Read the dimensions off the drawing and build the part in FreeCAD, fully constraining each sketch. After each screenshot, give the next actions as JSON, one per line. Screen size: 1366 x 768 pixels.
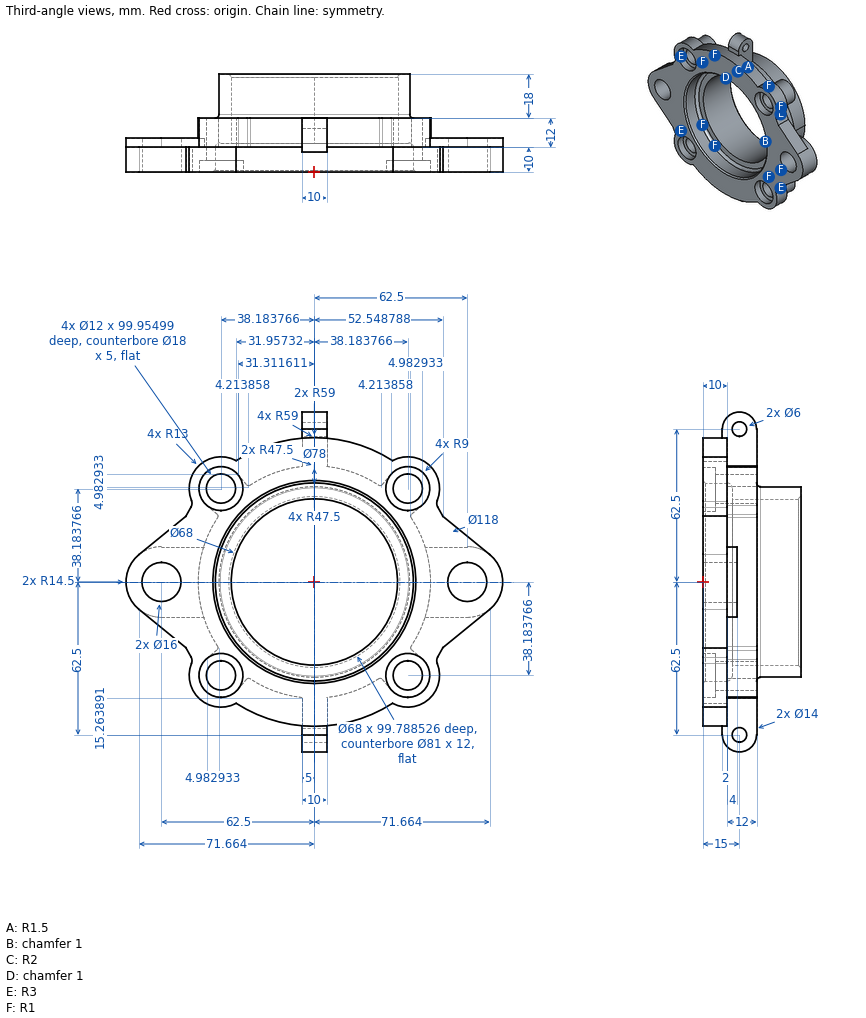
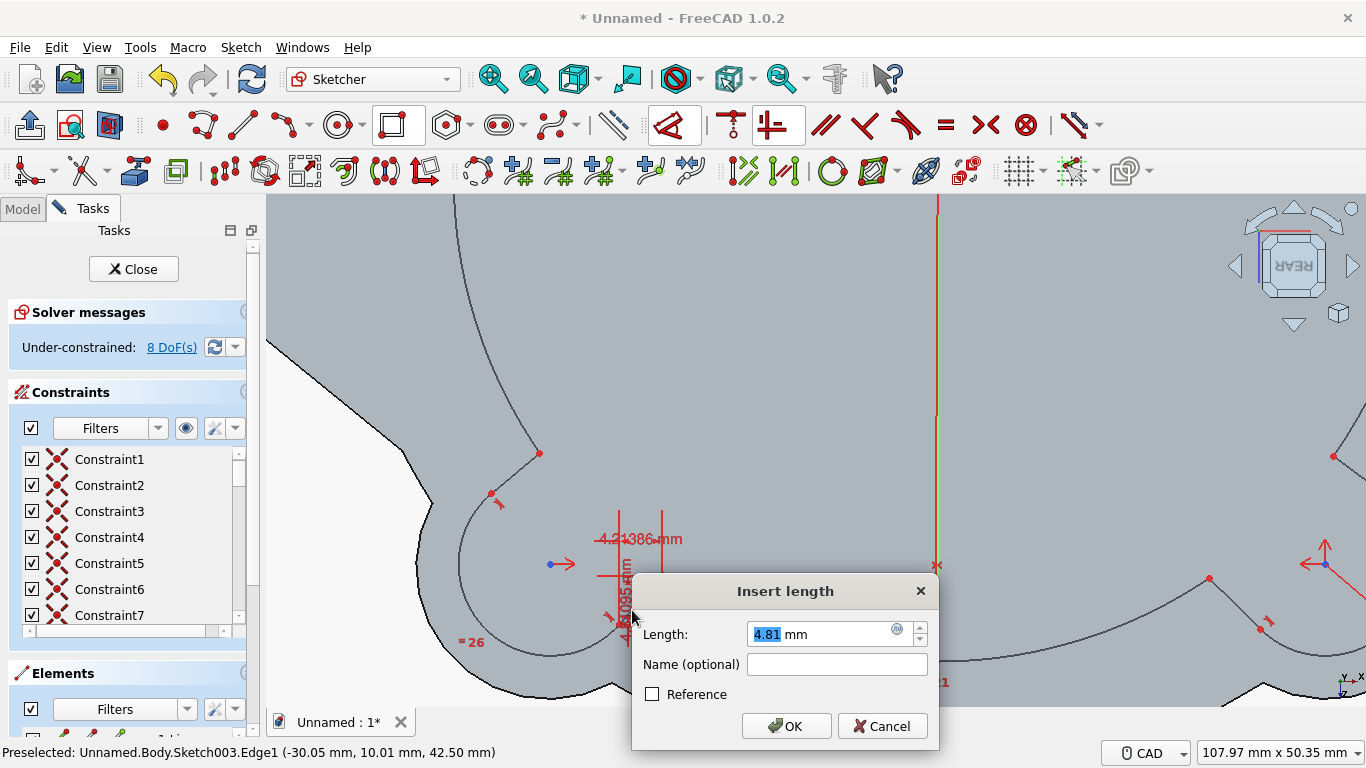
{"action": "type", "text": "4.982933"}
{"action": "key", "text": "Return"}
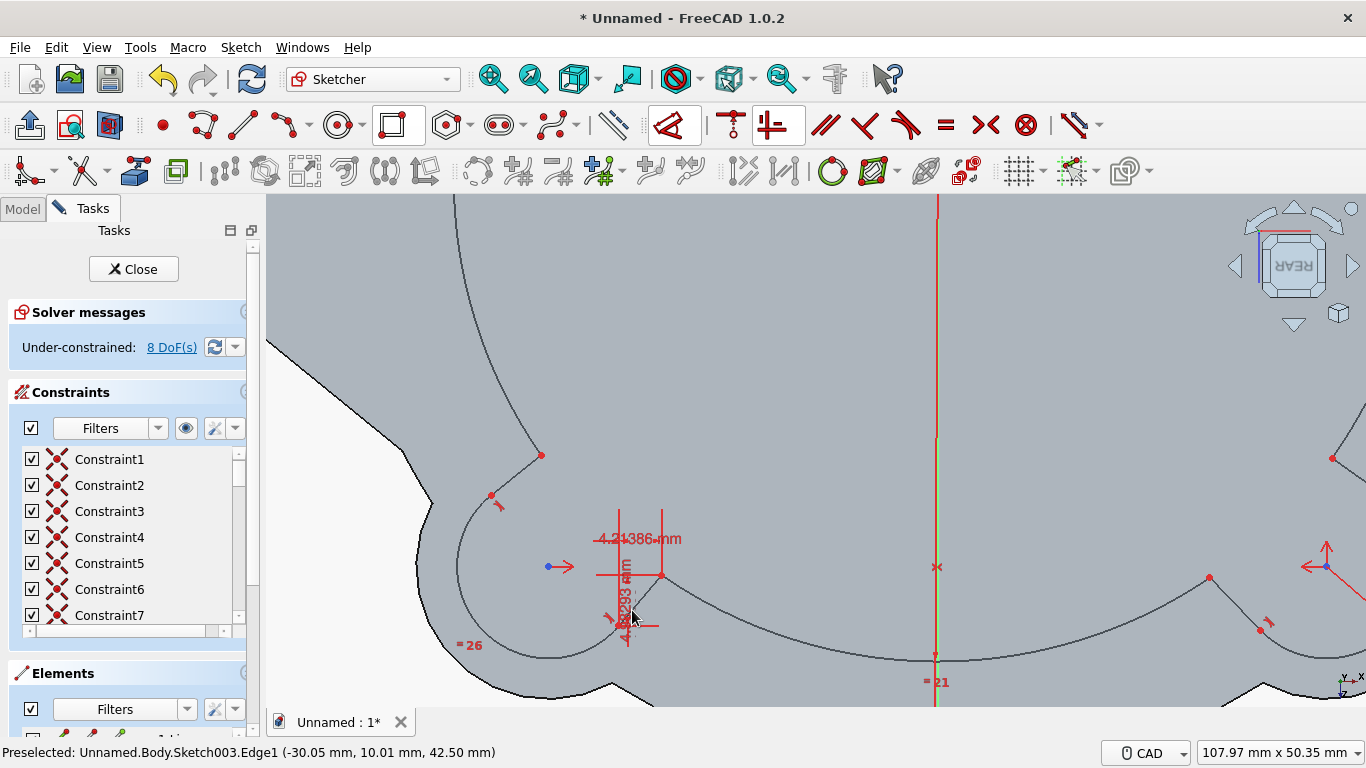
{"action": "scroll", "coordinate": [637, 609], "scroll_direction": "down", "scroll_amount": 5}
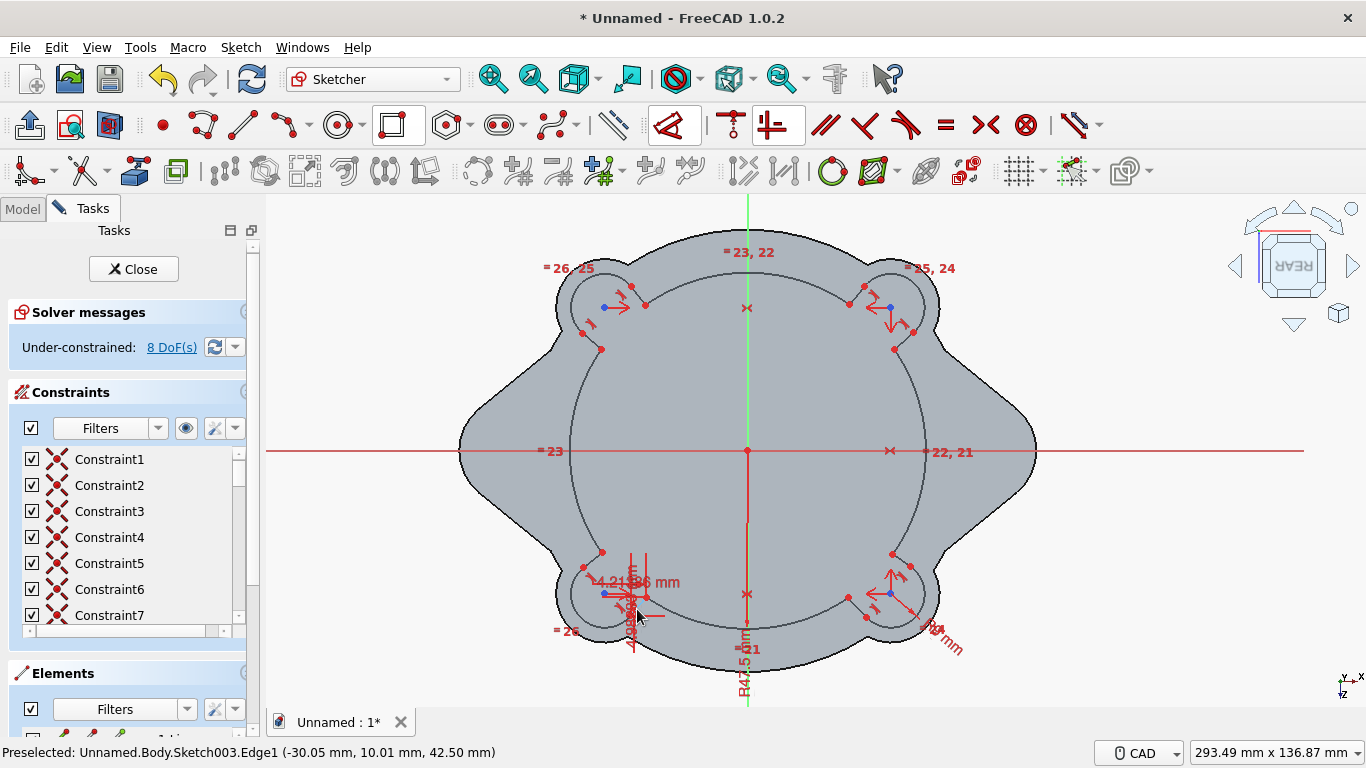
{"action": "scroll", "coordinate": [854, 604], "scroll_direction": "up", "scroll_amount": 5}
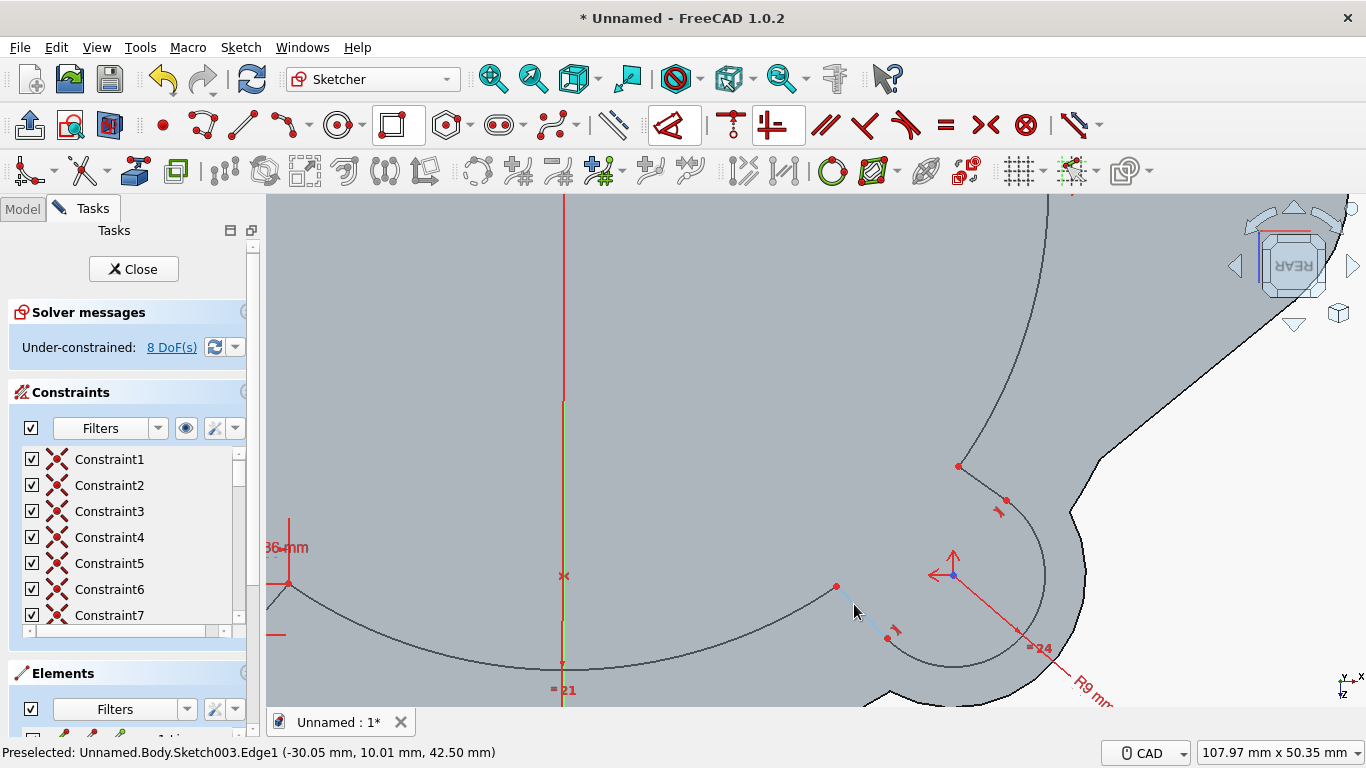
{"action": "left_click", "coordinate": [852, 602]}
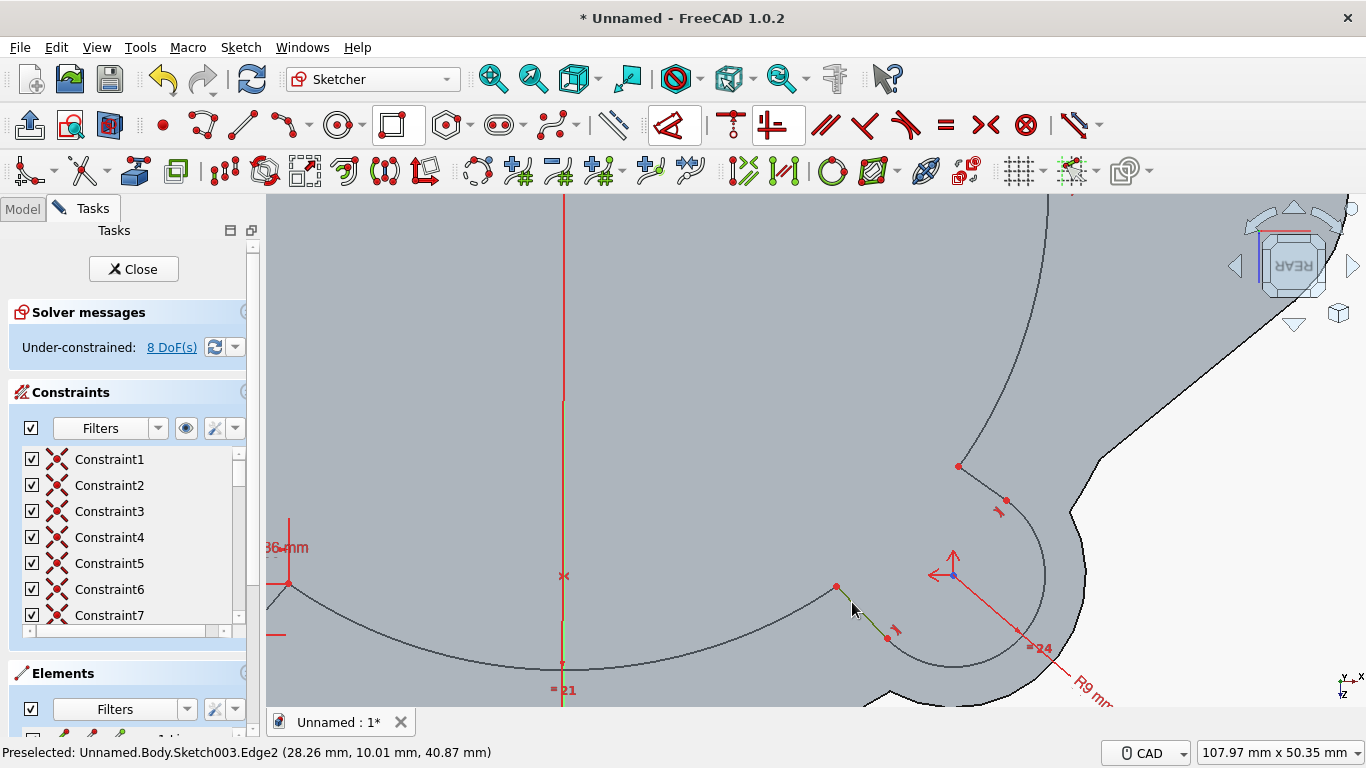
{"action": "left_click", "coordinate": [696, 126]}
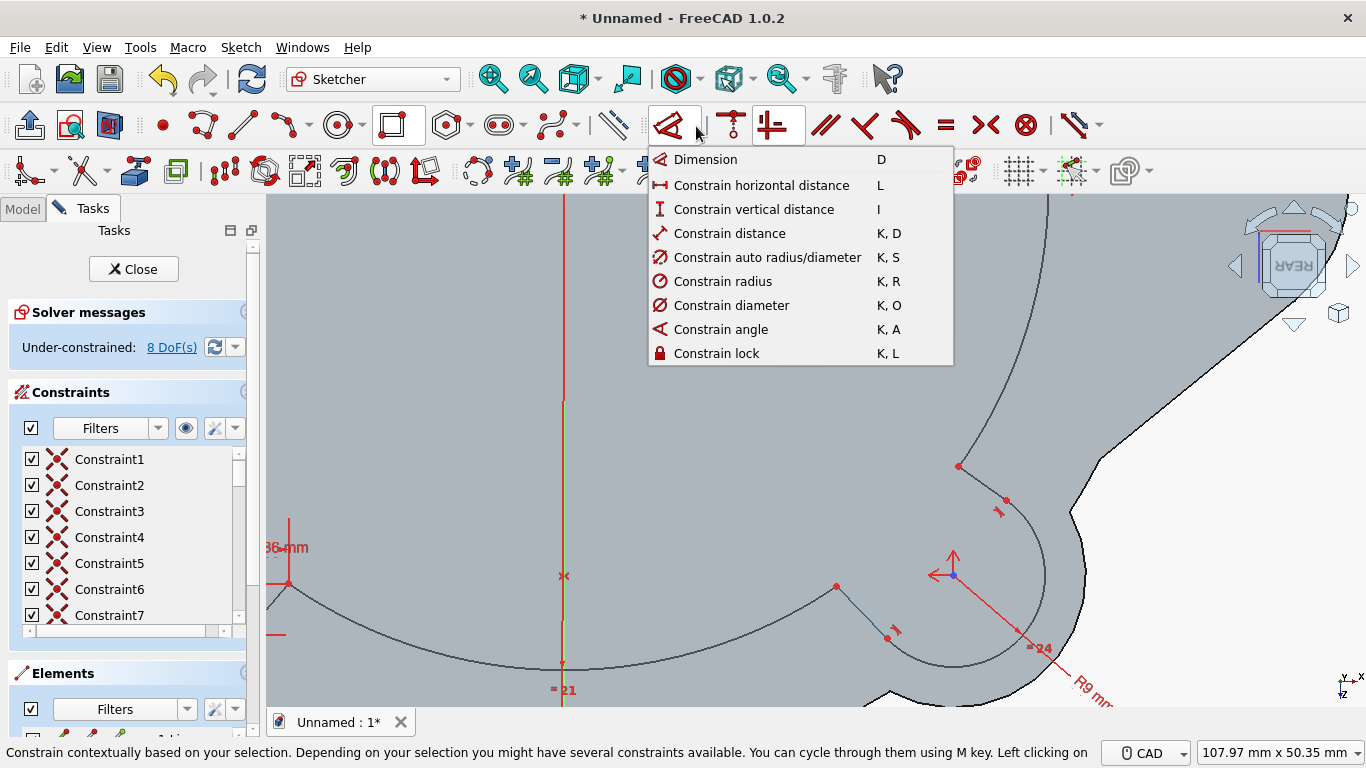
{"action": "left_click", "coordinate": [801, 185]}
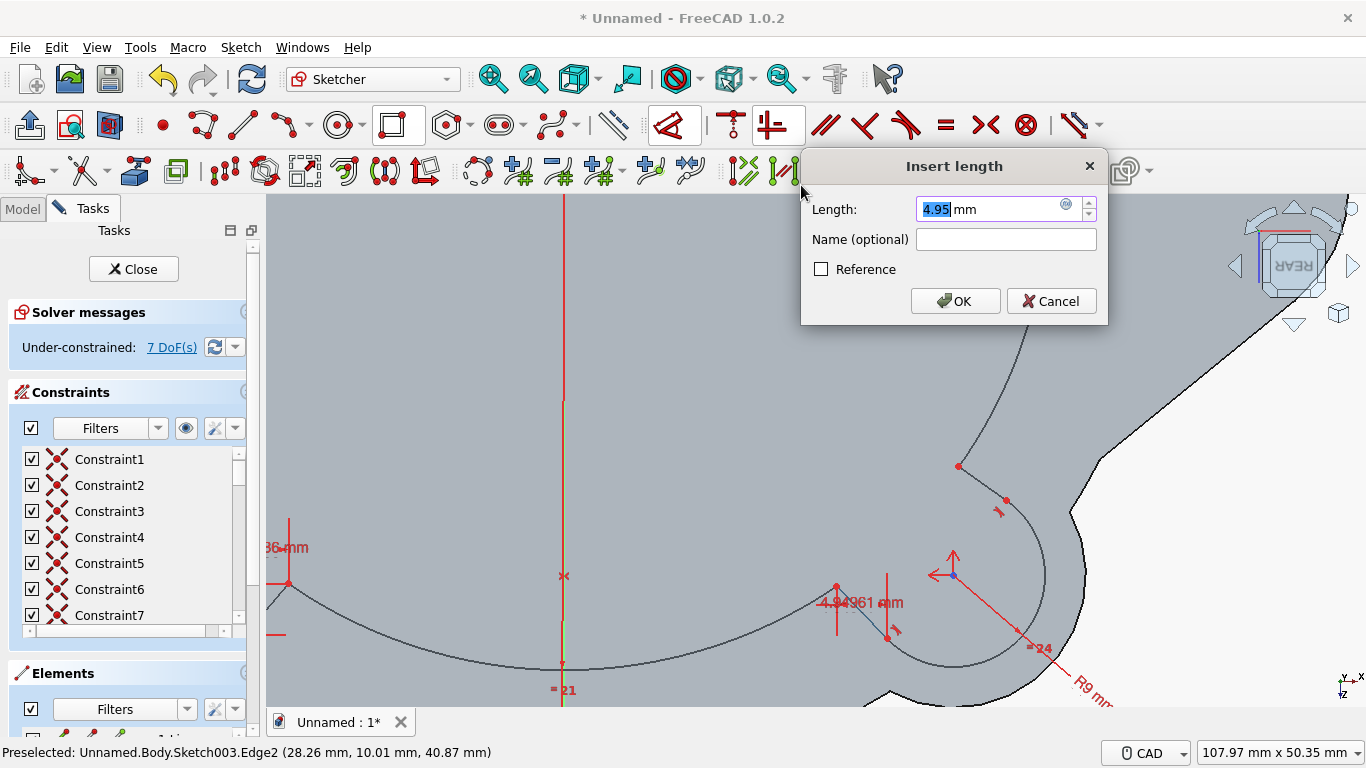
{"action": "type", "text": "4.213858"}
{"action": "key", "text": "Return"}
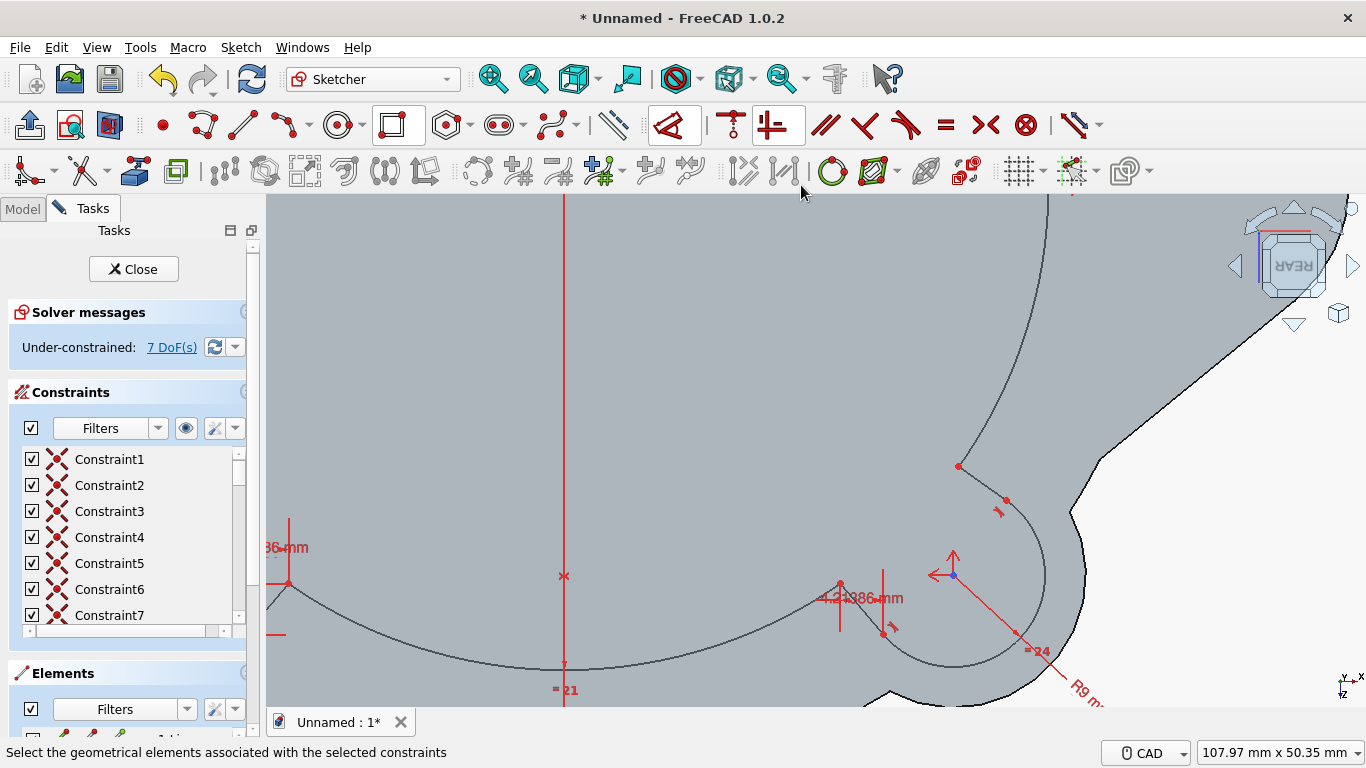
{"action": "left_click", "coordinate": [992, 490]}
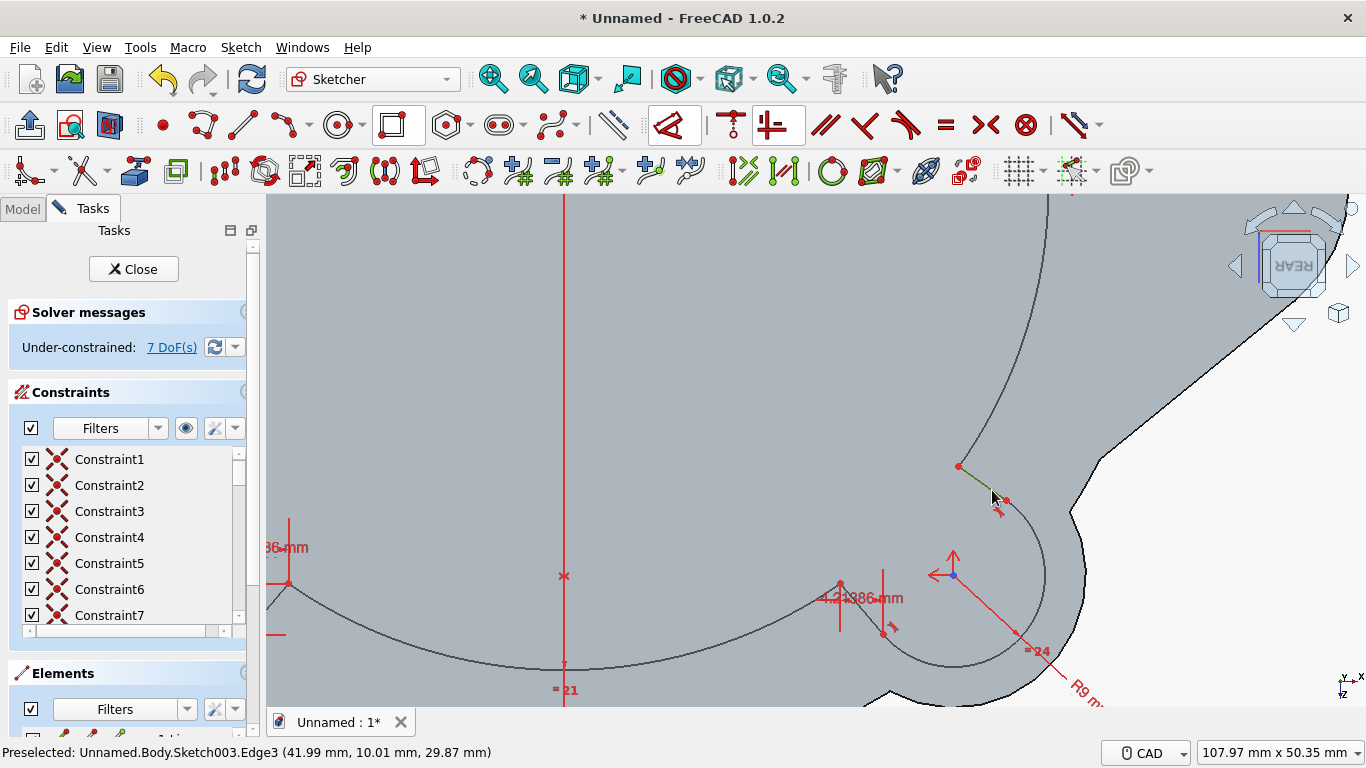
{"action": "left_click", "coordinate": [696, 126]}